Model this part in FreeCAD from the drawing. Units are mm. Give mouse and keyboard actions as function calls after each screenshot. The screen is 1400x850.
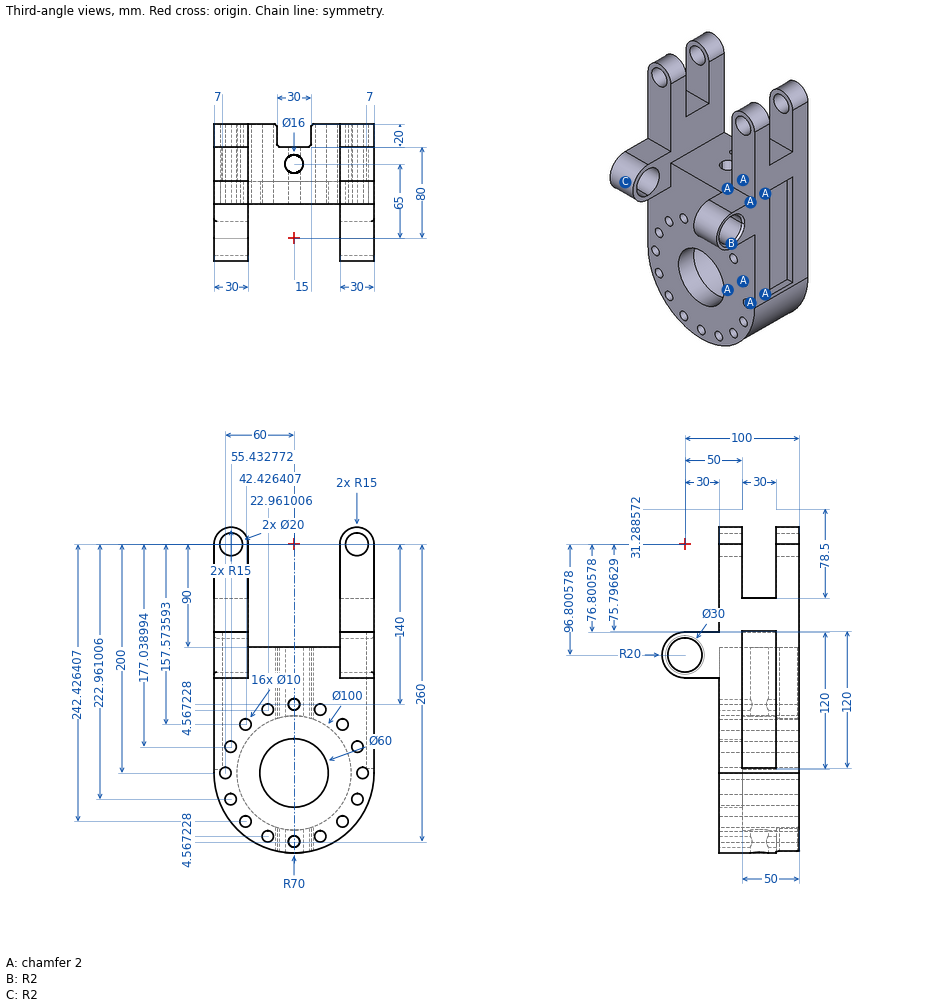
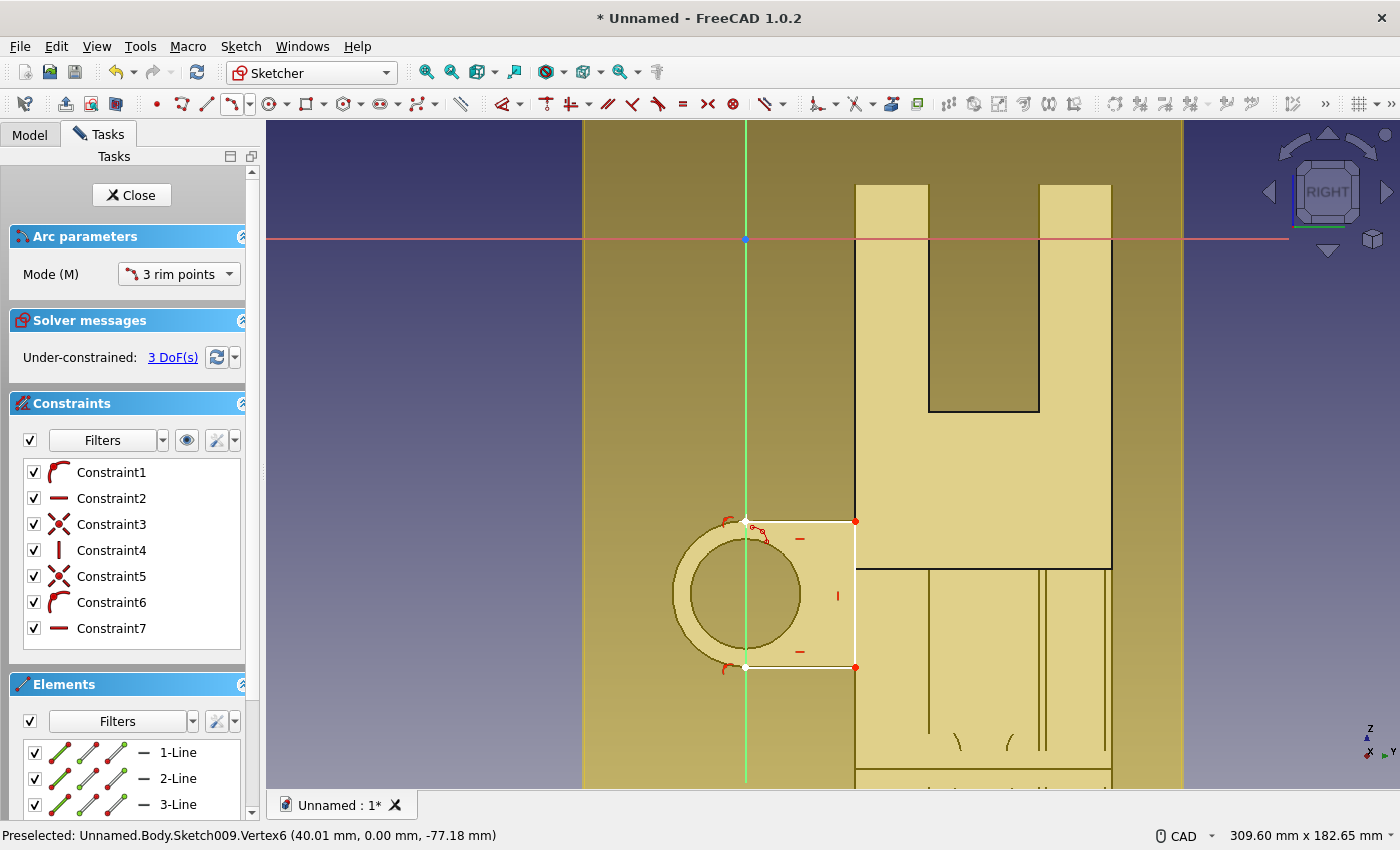
click(746, 522)
click(746, 668)
click(672, 594)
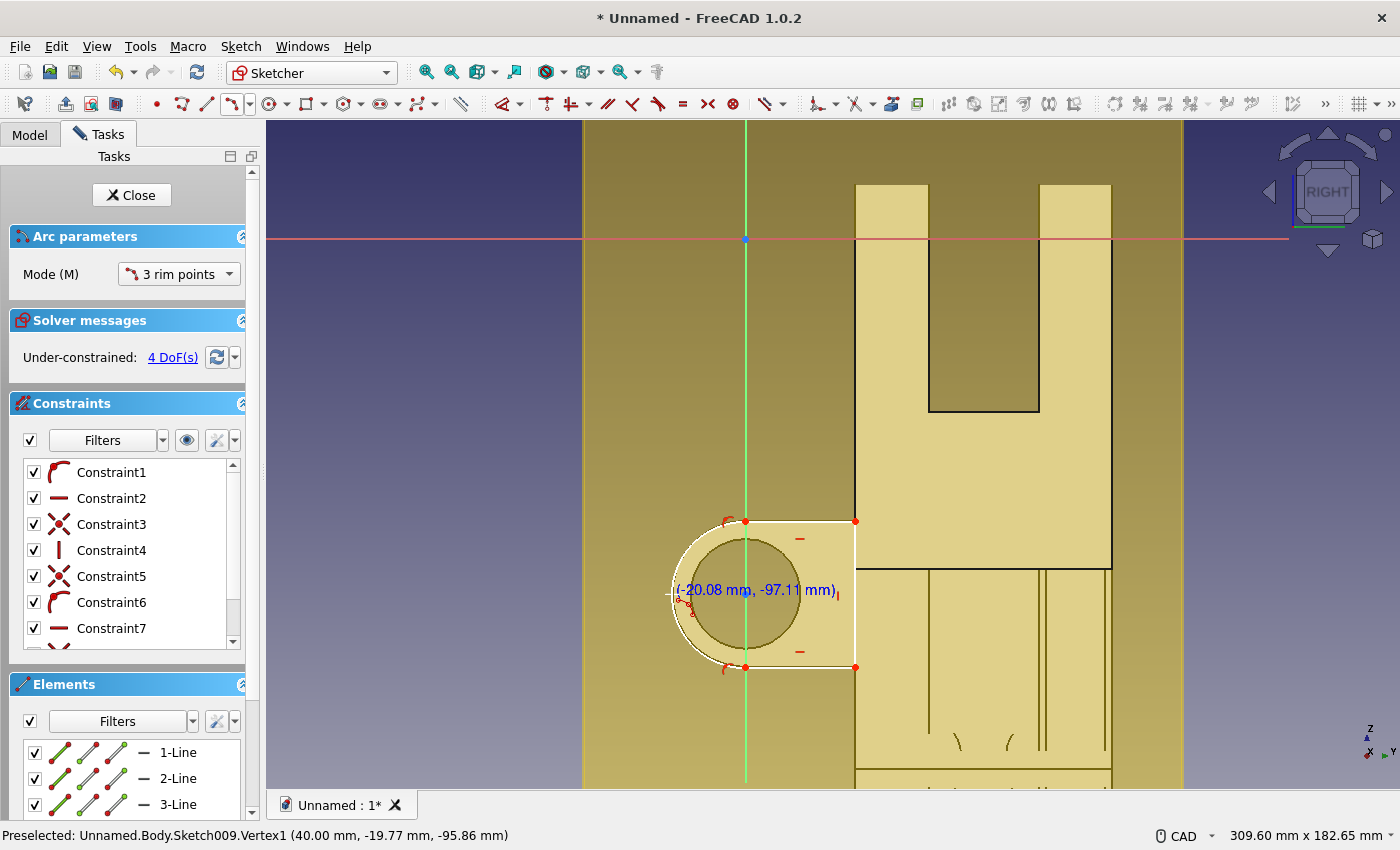
key(g)
key(c)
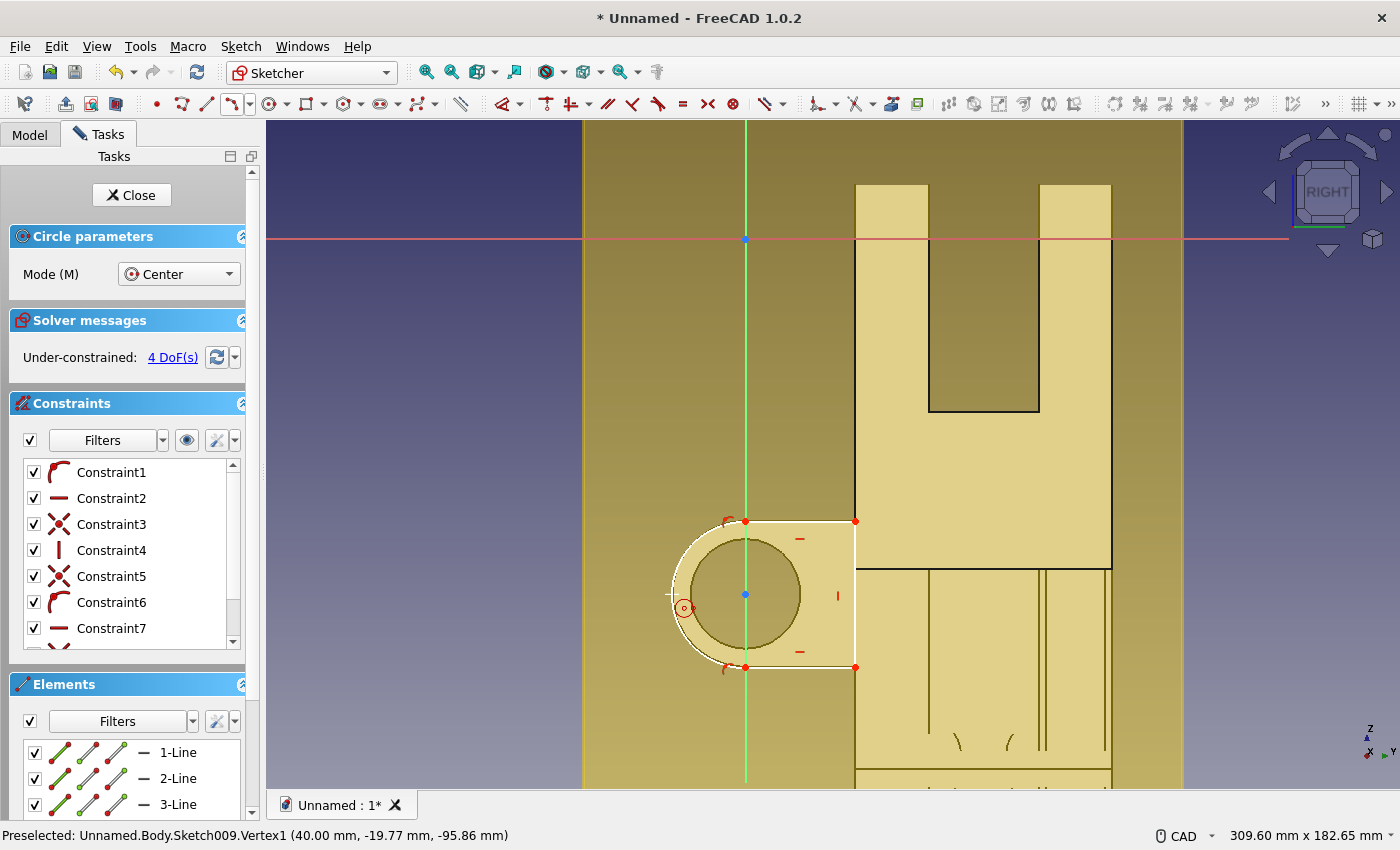
click(746, 594)
click(784, 555)
key(Escape)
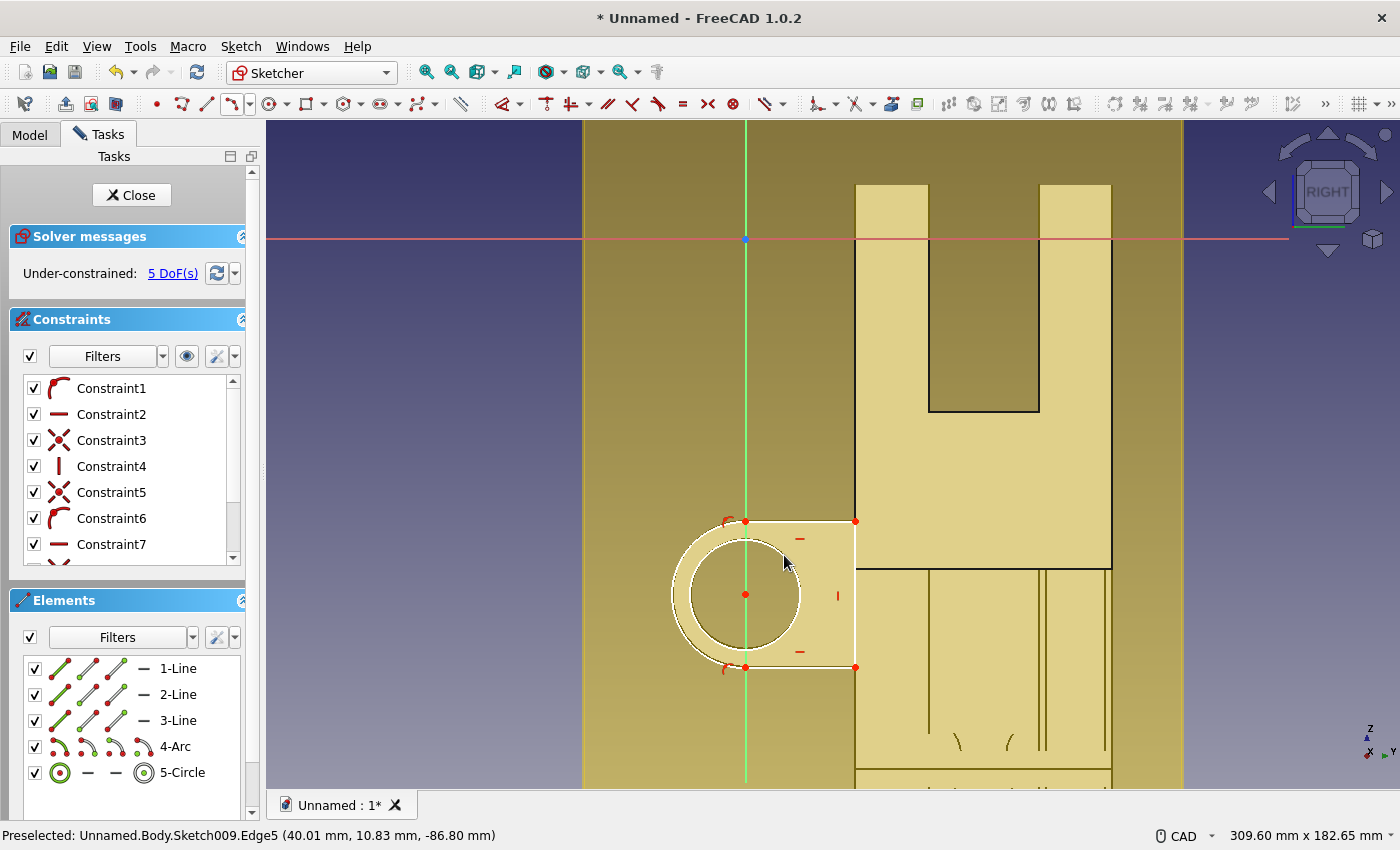
click(778, 668)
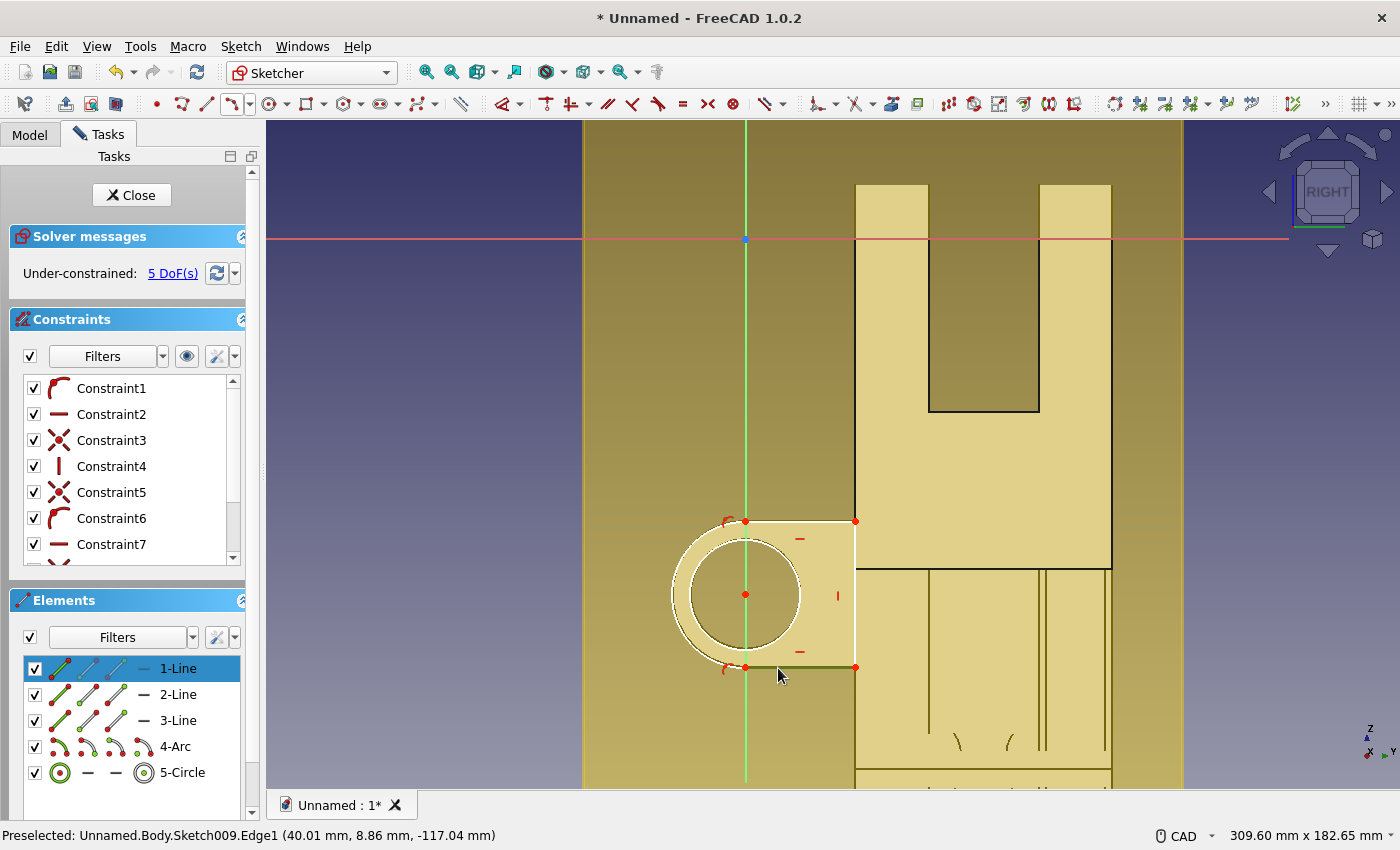
click(686, 552)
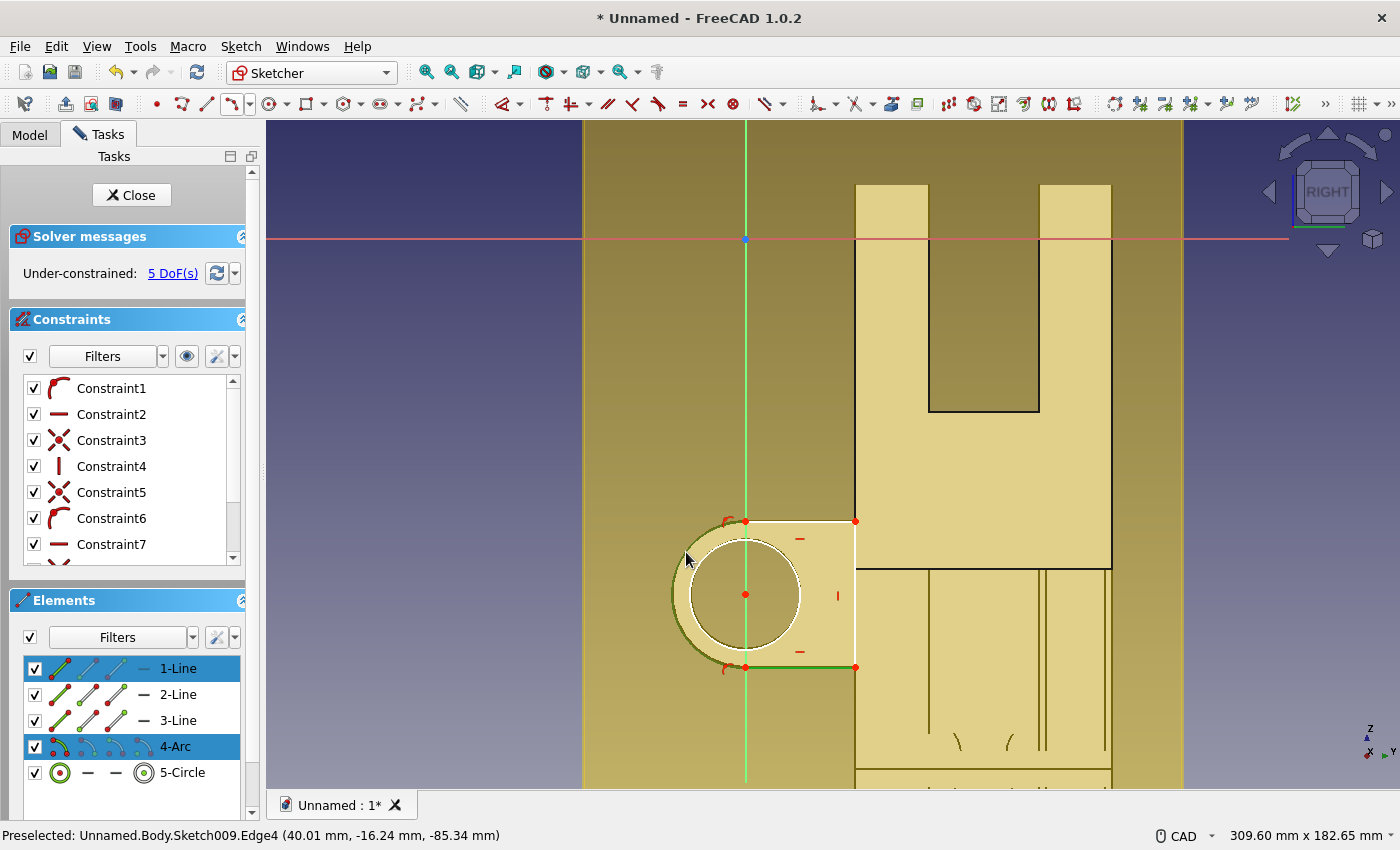
key(t)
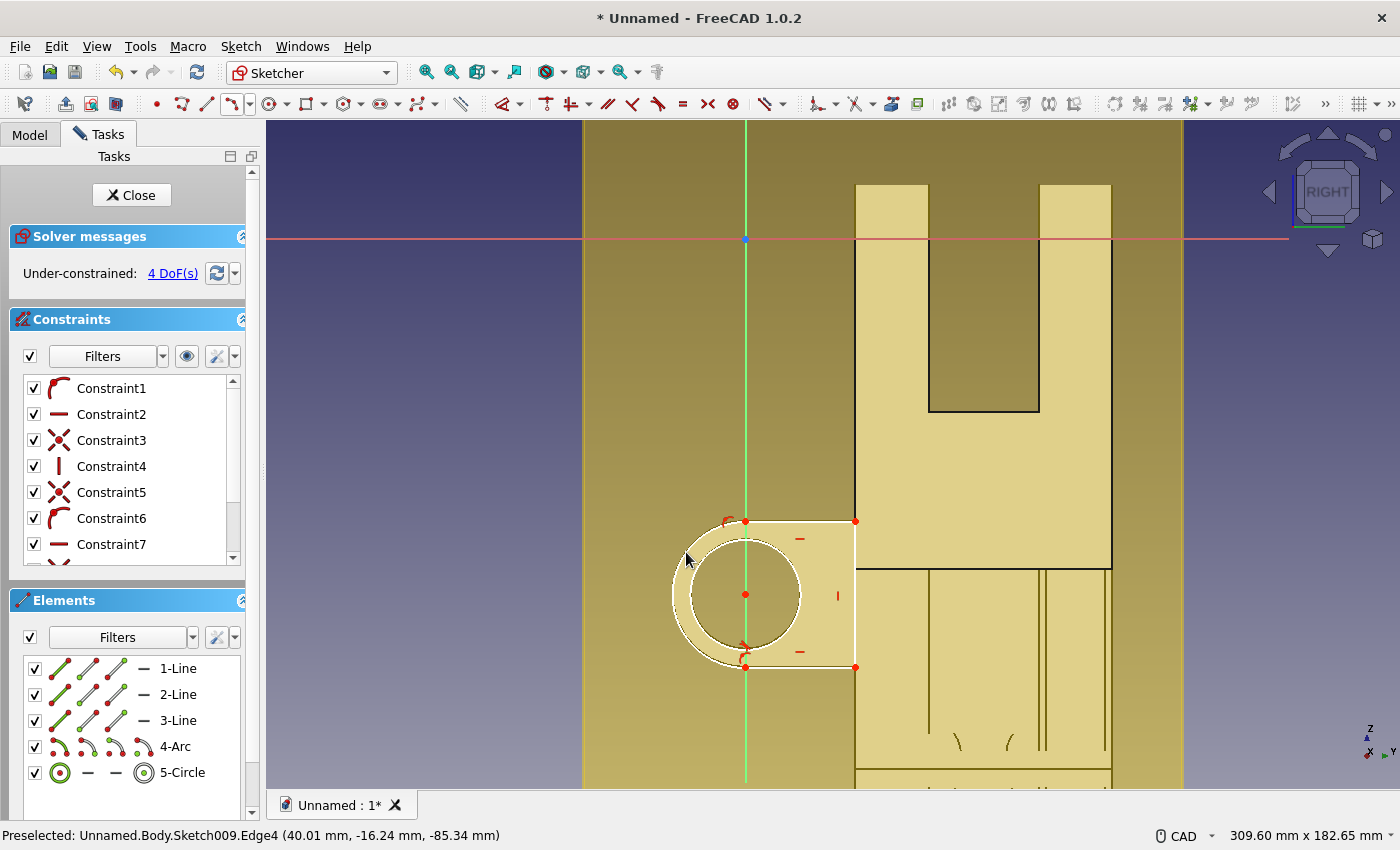
key(d)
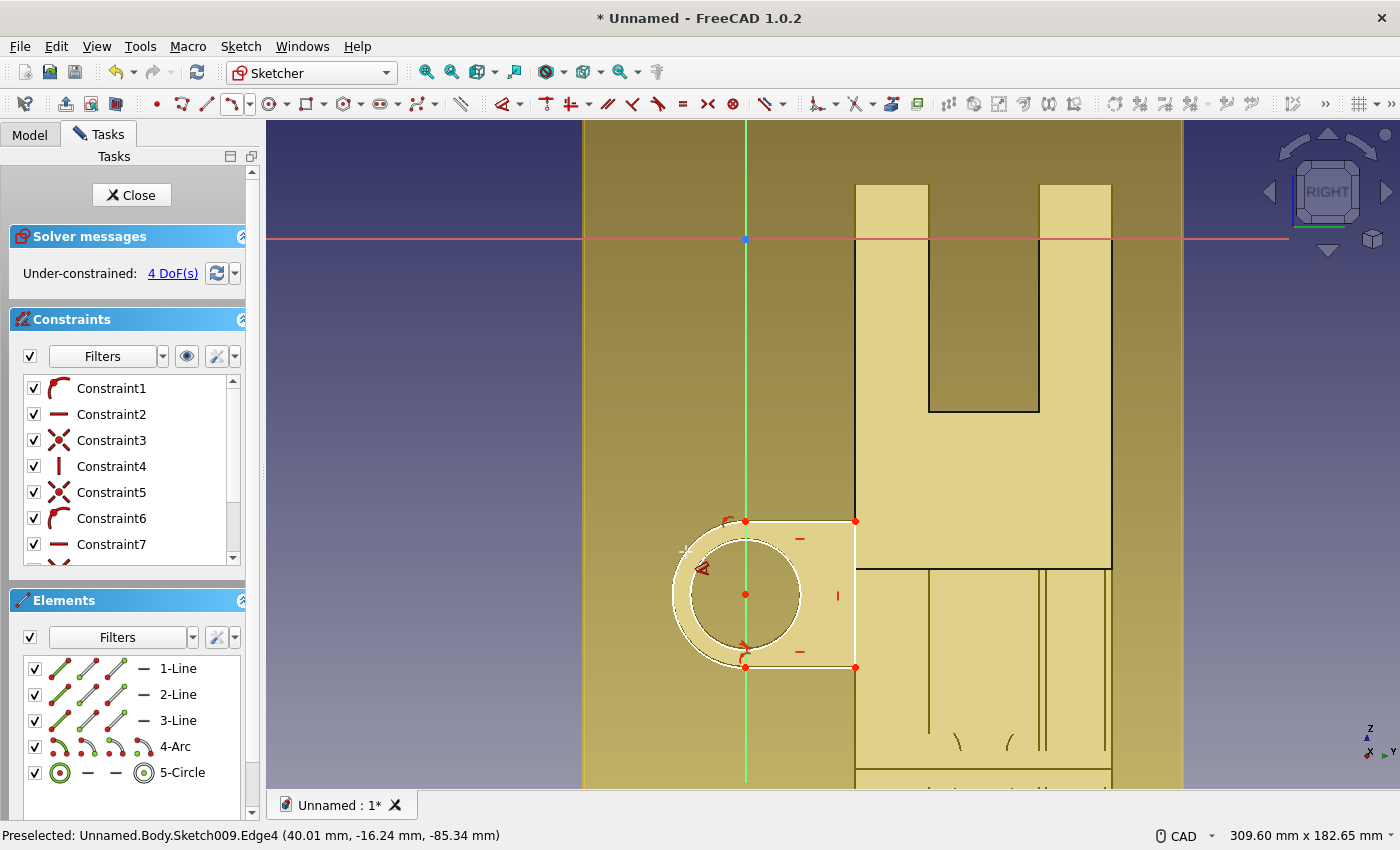
click(686, 552)
click(660, 533)